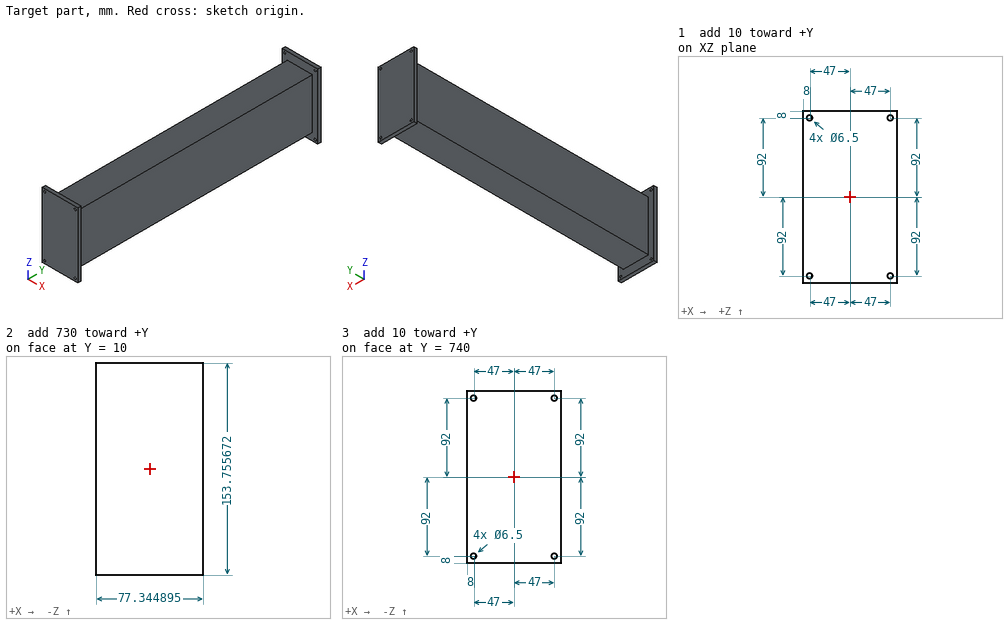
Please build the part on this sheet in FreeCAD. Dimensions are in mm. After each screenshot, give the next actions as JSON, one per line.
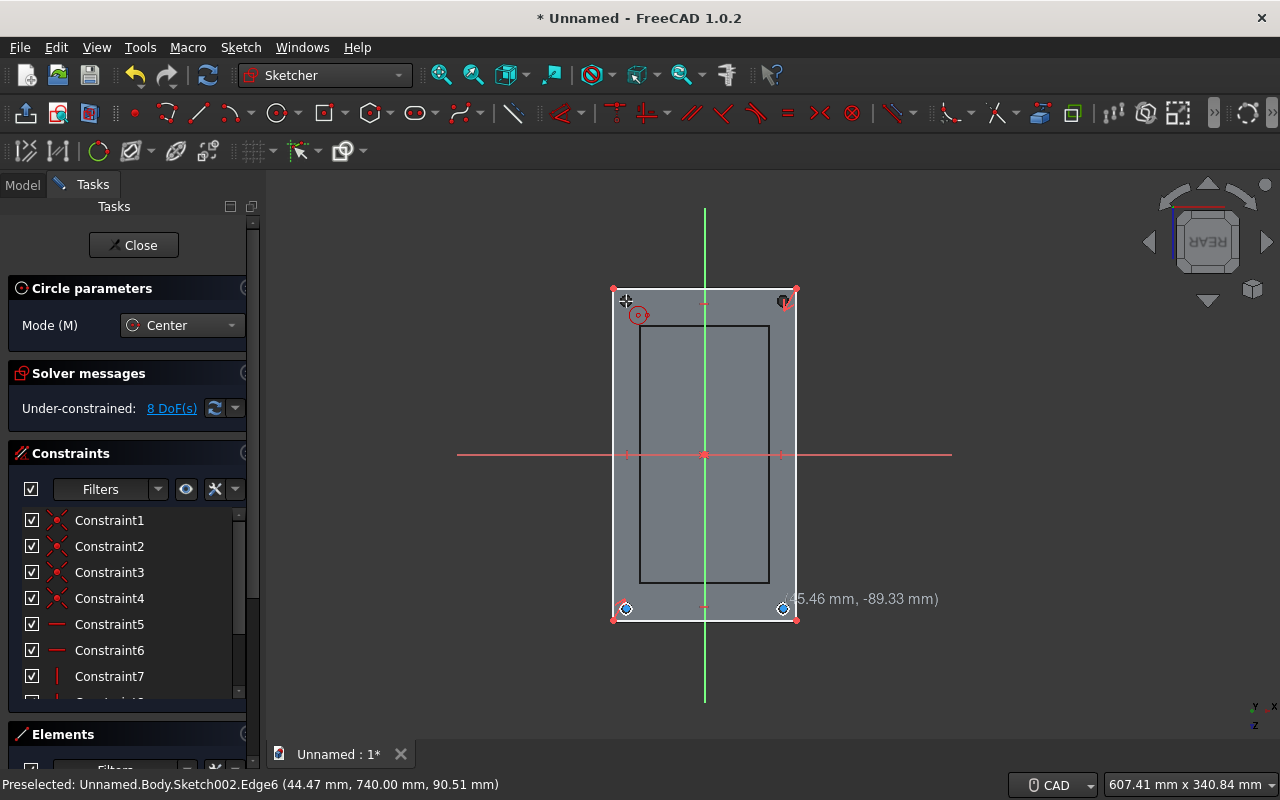
{"action": "left_click", "coordinate": [626, 301]}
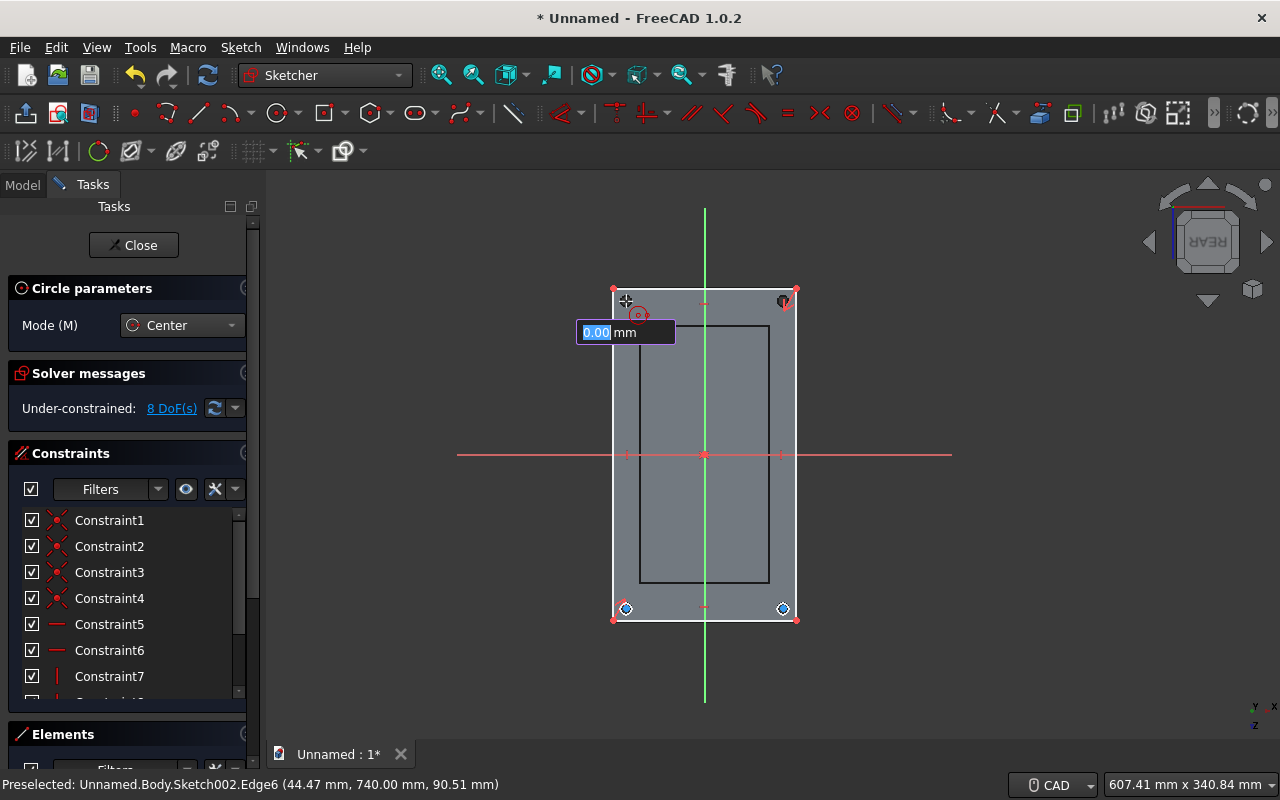
{"action": "scroll", "coordinate": [630, 305], "scroll_direction": "up", "scroll_amount": 6}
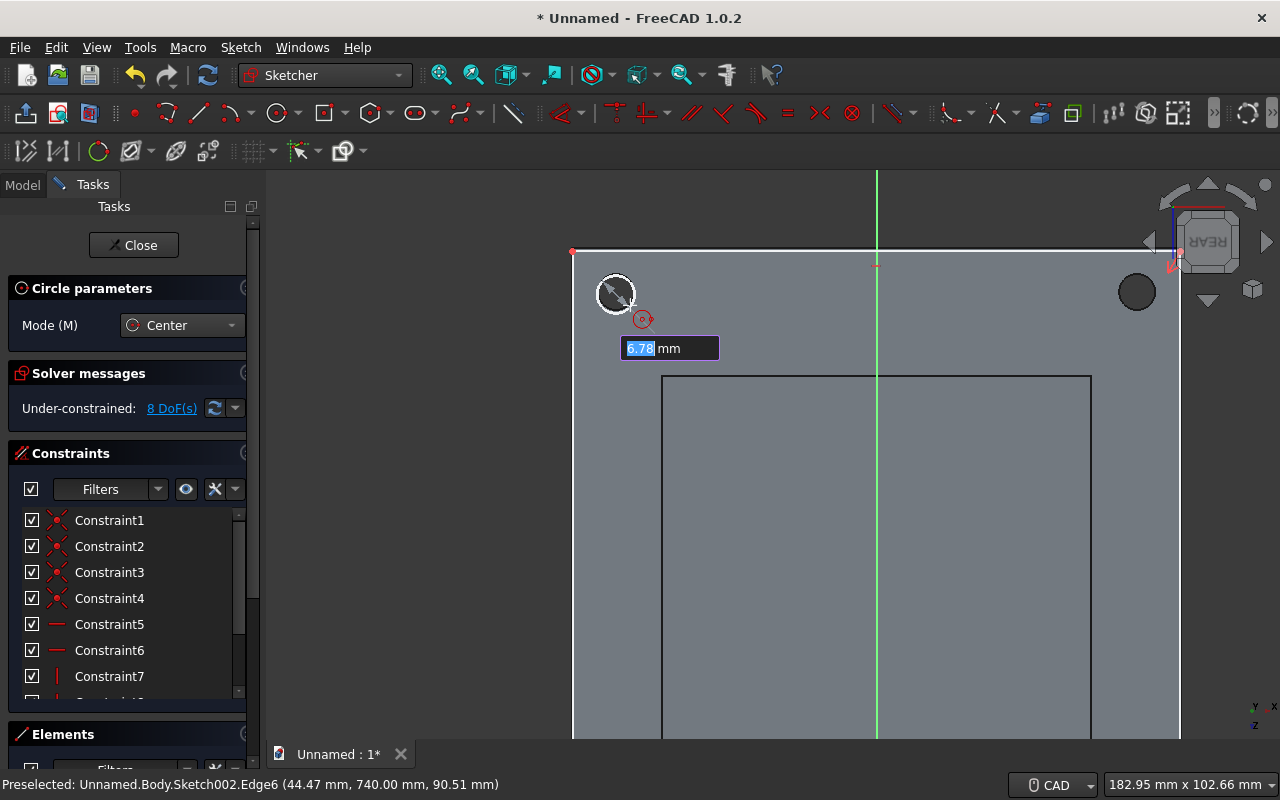
{"action": "left_click", "coordinate": [629, 305]}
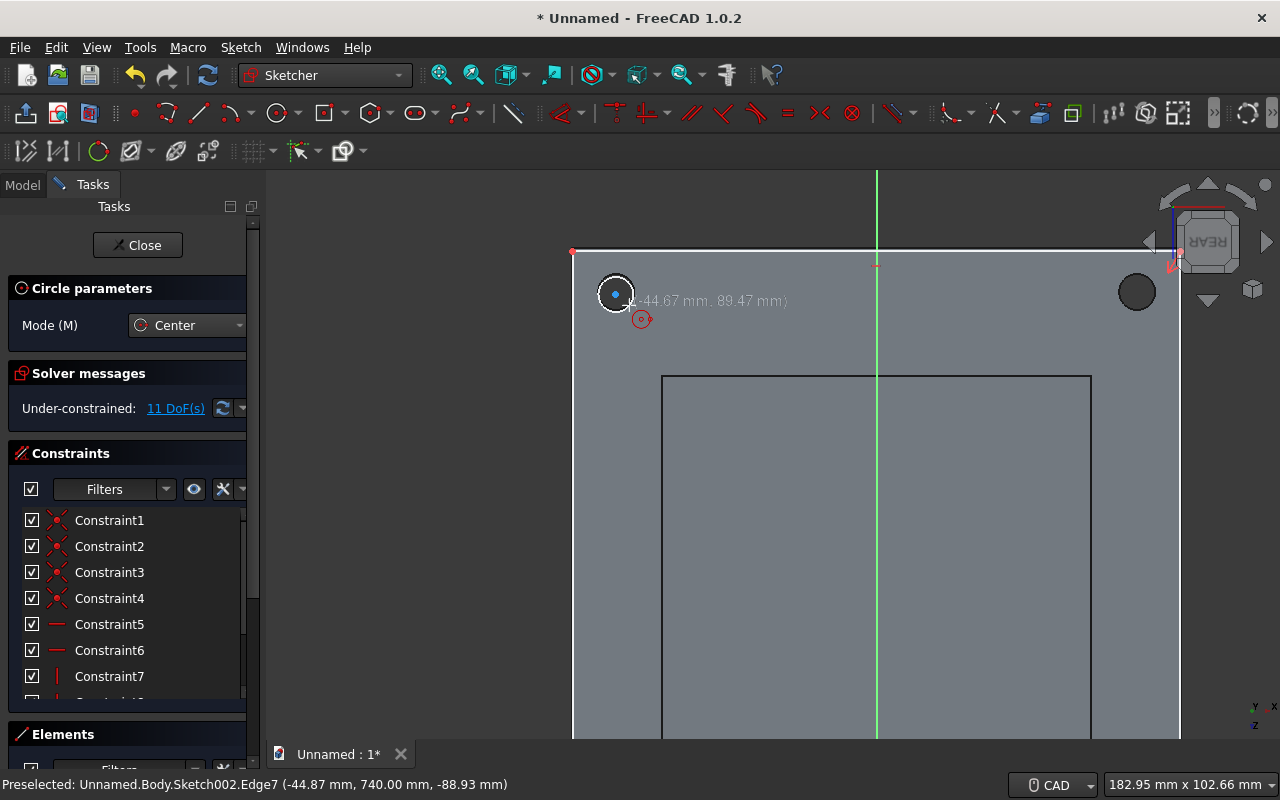
{"action": "scroll", "coordinate": [630, 305], "scroll_direction": "down", "scroll_amount": 6}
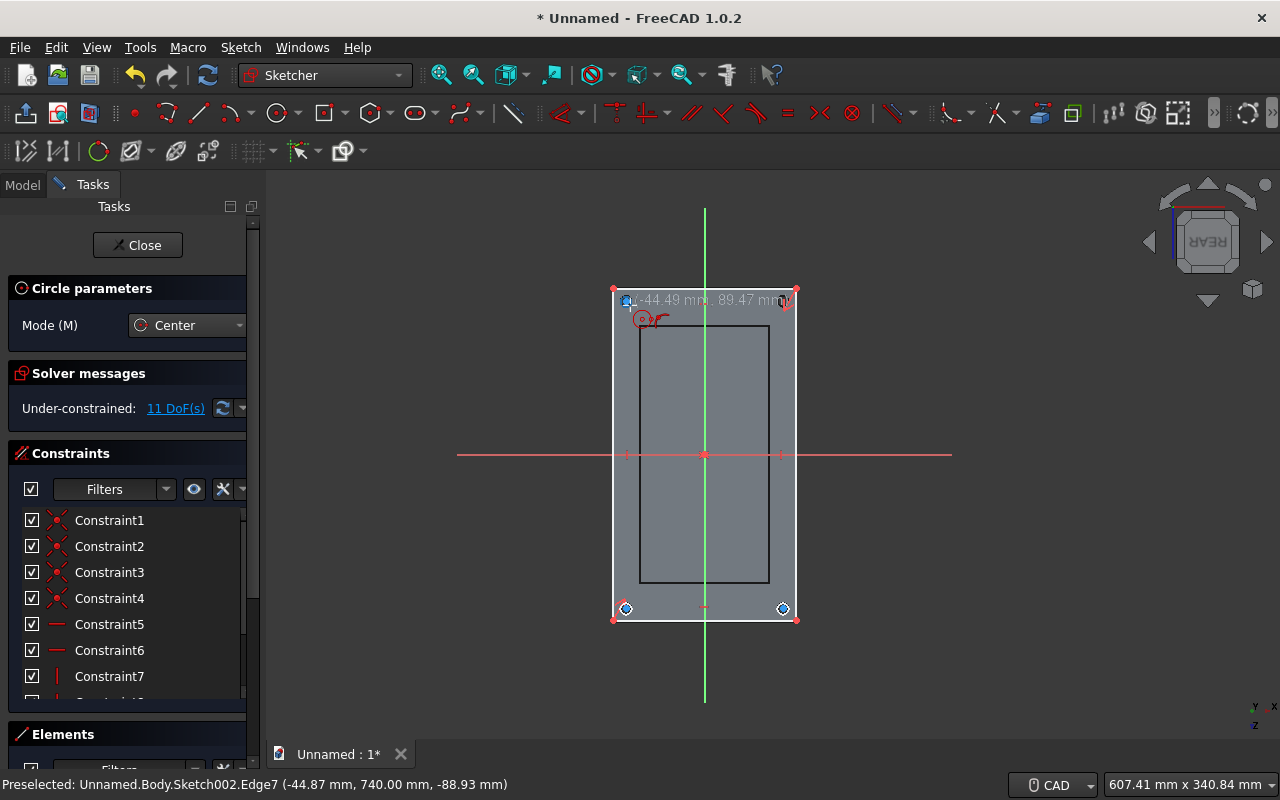
{"action": "scroll", "coordinate": [783, 301], "scroll_direction": "up", "scroll_amount": 8}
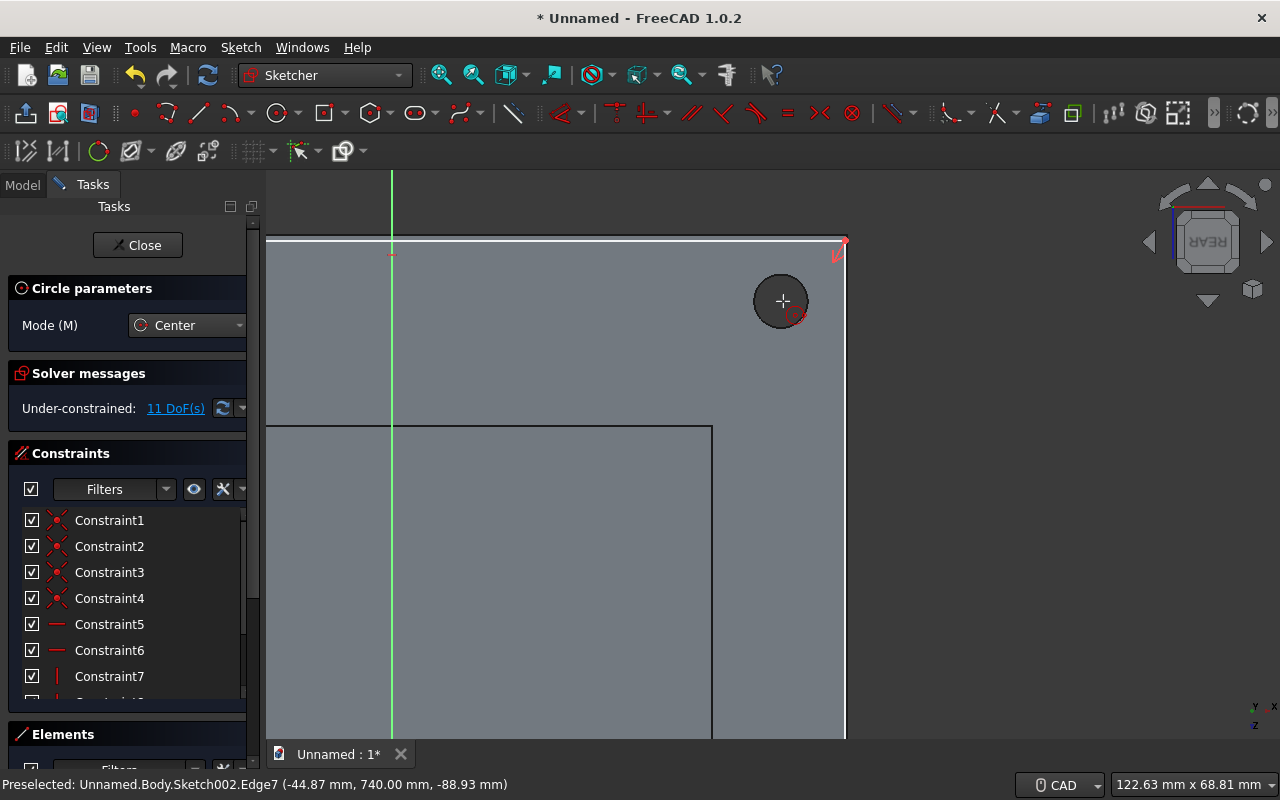
{"action": "scroll", "coordinate": [783, 301], "scroll_direction": "down", "scroll_amount": 8}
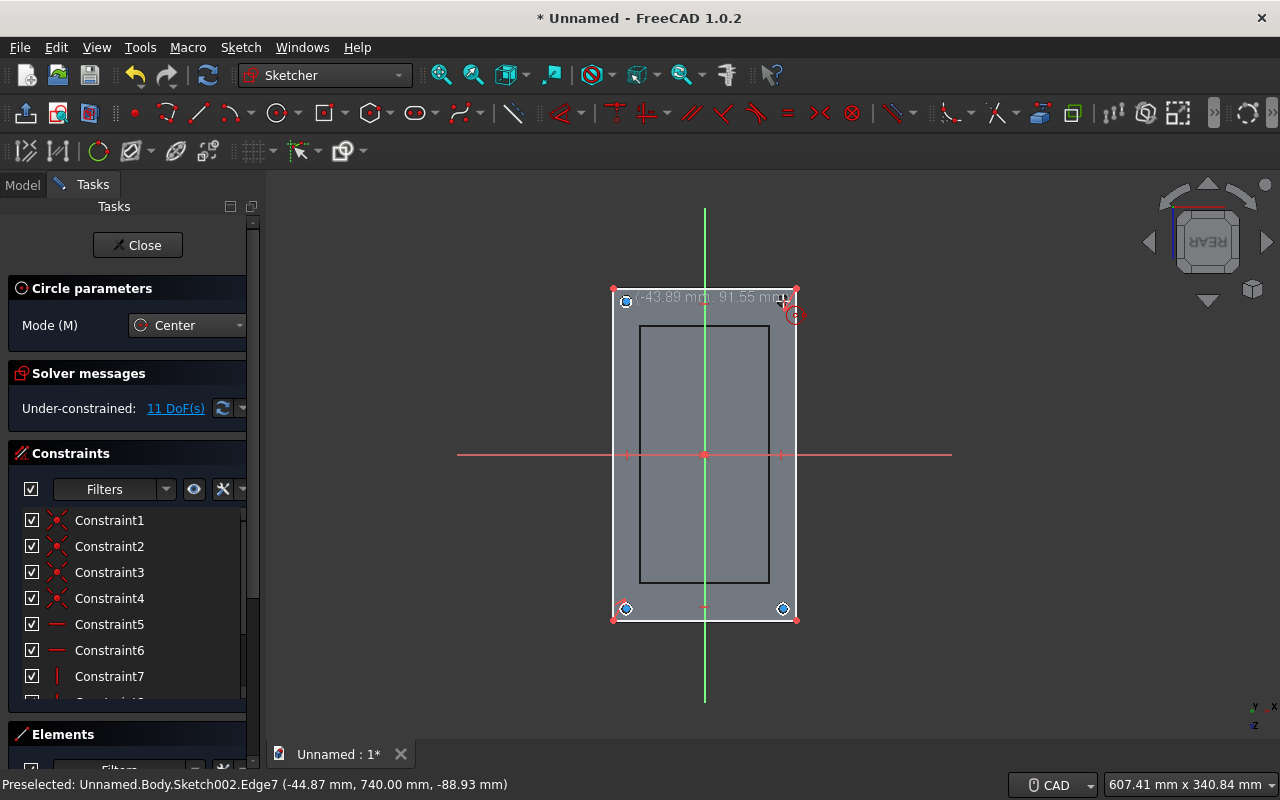
{"action": "left_click", "coordinate": [783, 301]}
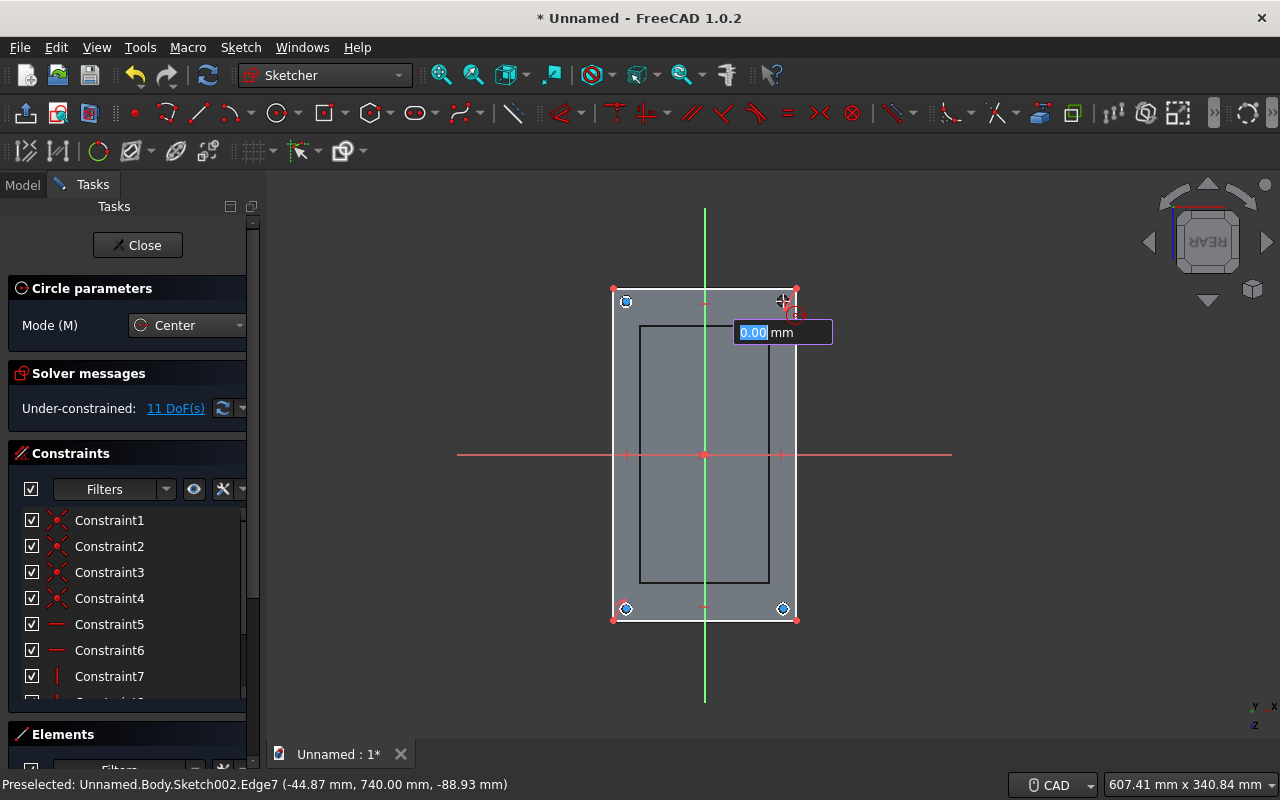
{"action": "scroll", "coordinate": [779, 305], "scroll_direction": "up", "scroll_amount": 6}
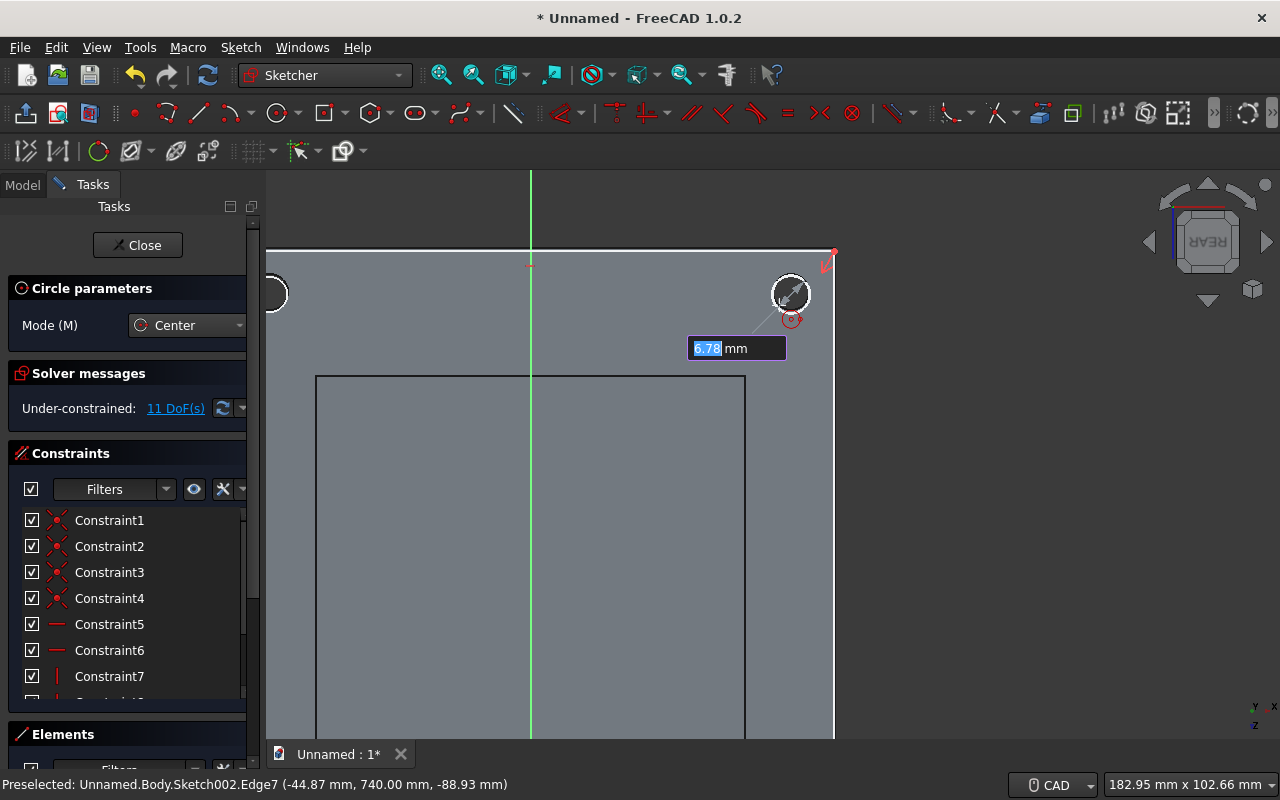
{"action": "left_click", "coordinate": [778, 305]}
{"action": "key", "text": "Escape"}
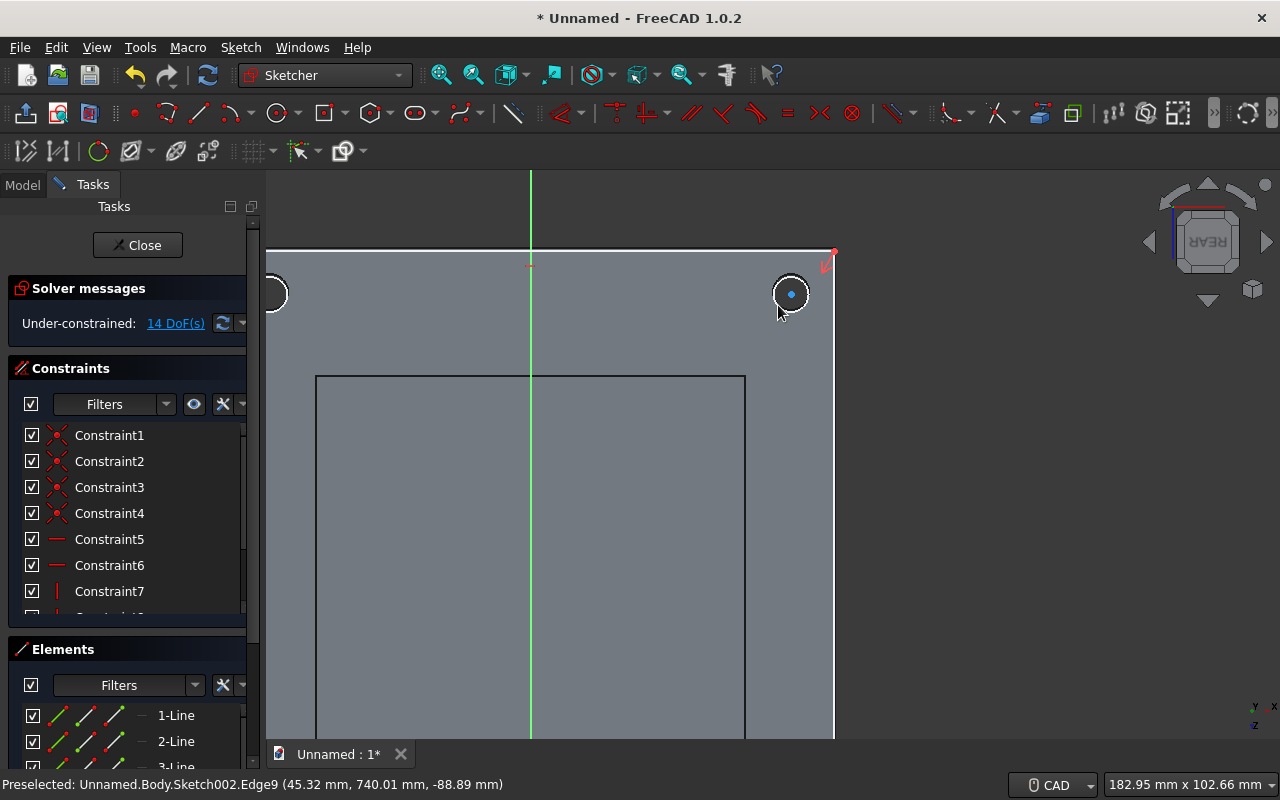
{"action": "scroll", "coordinate": [779, 305], "scroll_direction": "down", "scroll_amount": 6}